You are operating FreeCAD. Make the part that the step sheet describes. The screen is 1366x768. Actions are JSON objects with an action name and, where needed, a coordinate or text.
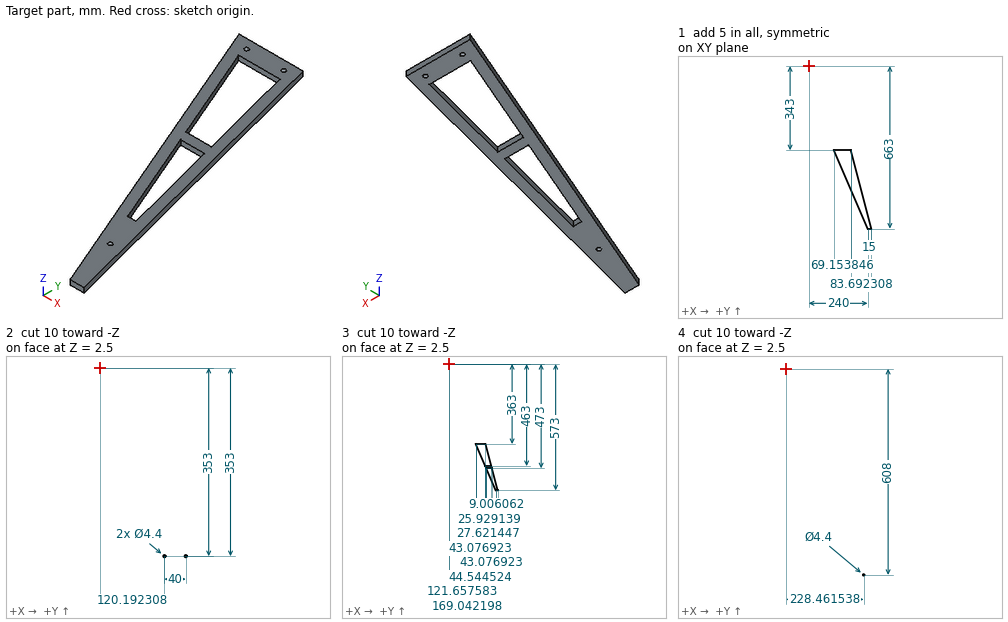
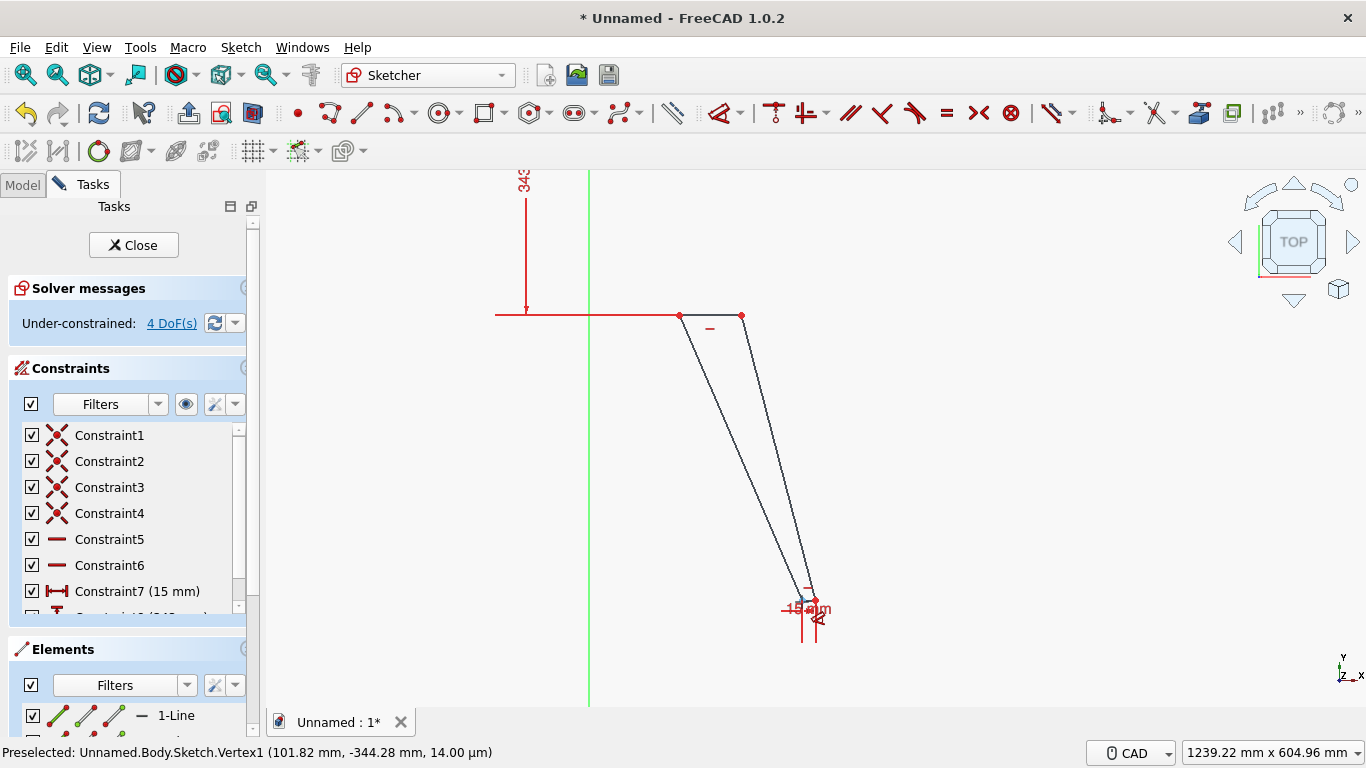
{"action": "left_click", "coordinate": [802, 601]}
{"action": "left_click", "coordinate": [696, 635]}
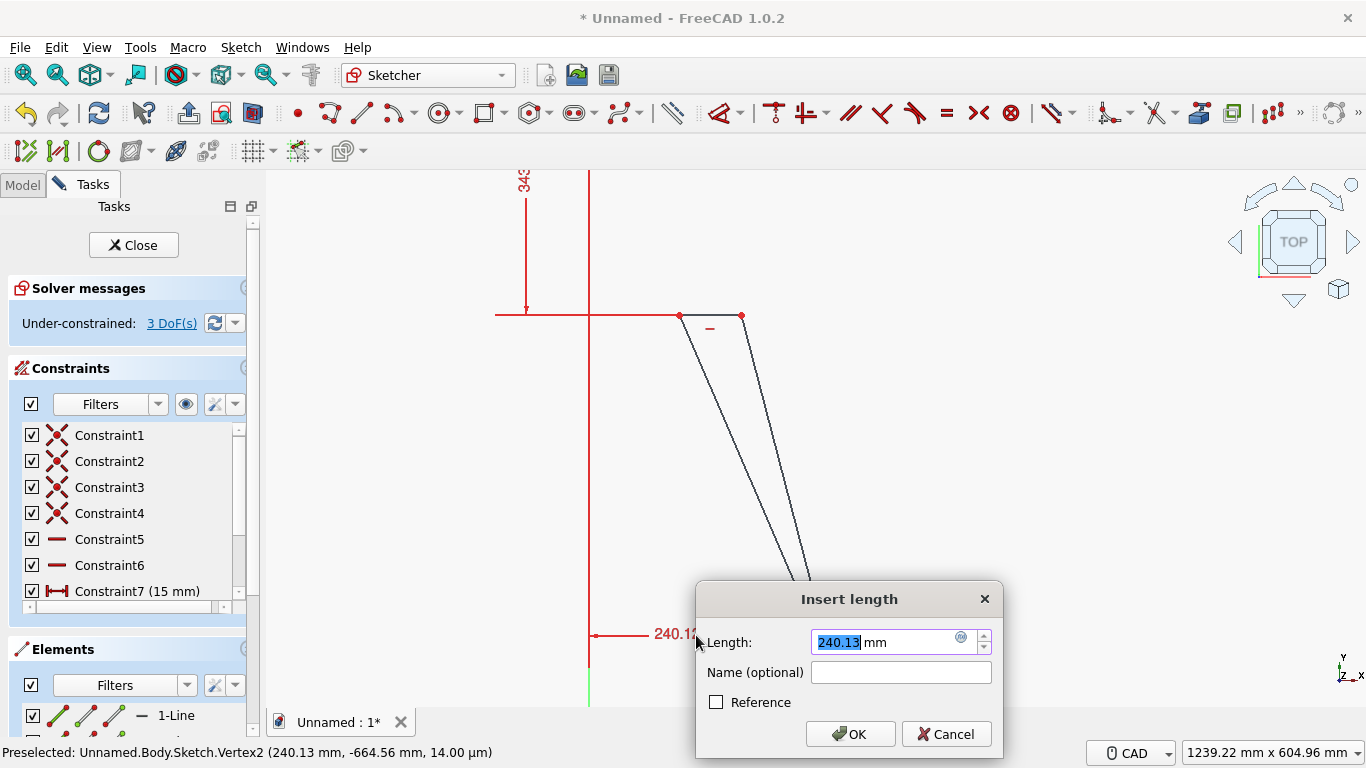
{"action": "type", "text": "240"}
{"action": "key", "text": "Return"}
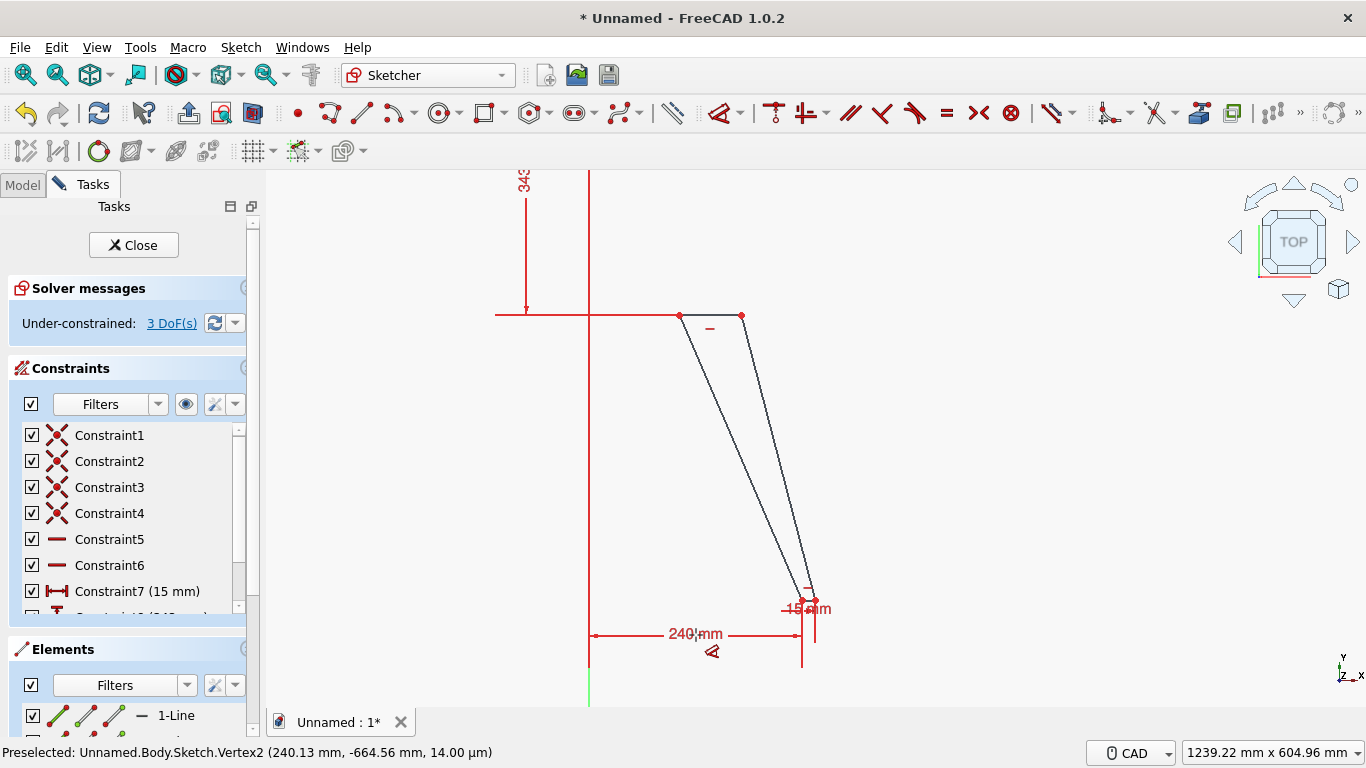
{"action": "left_click", "coordinate": [802, 601]}
{"action": "left_click", "coordinate": [555, 399]}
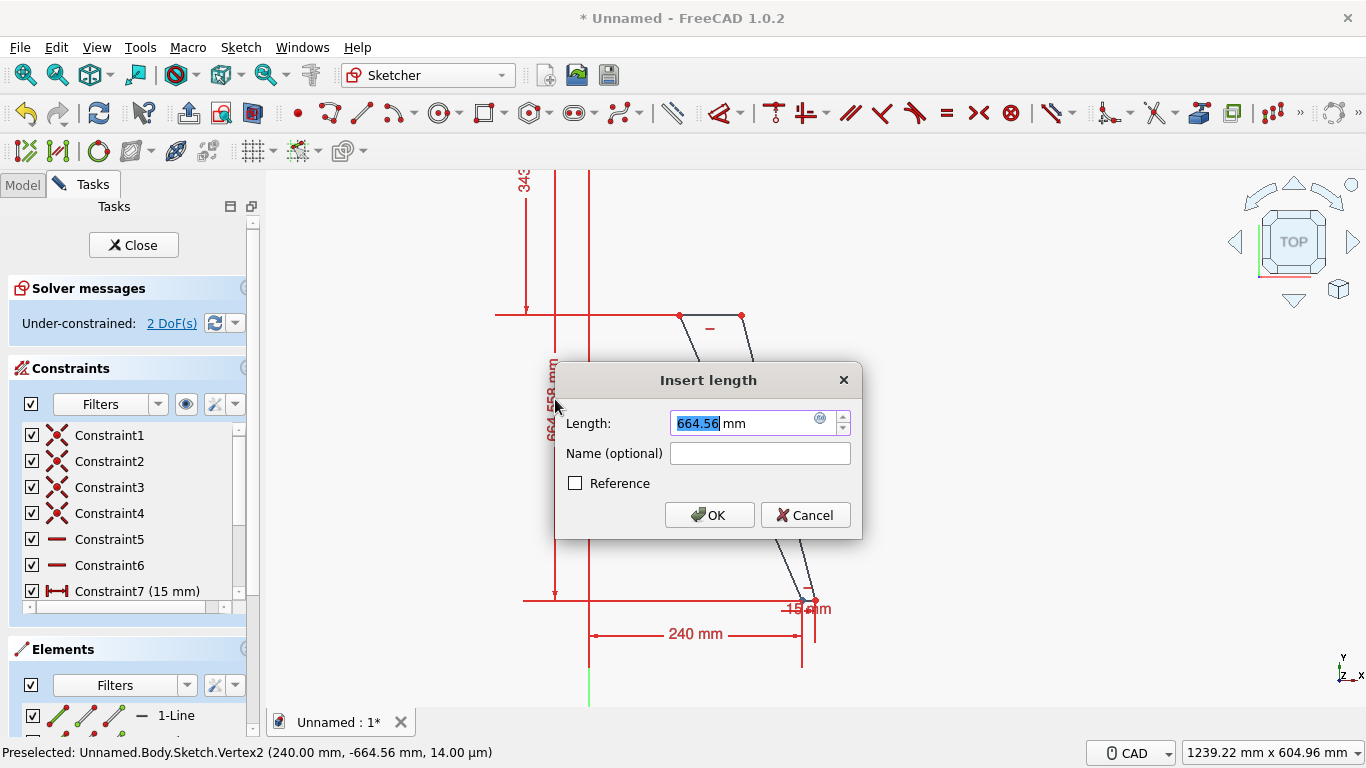
{"action": "type", "text": "663"}
{"action": "key", "text": "Return"}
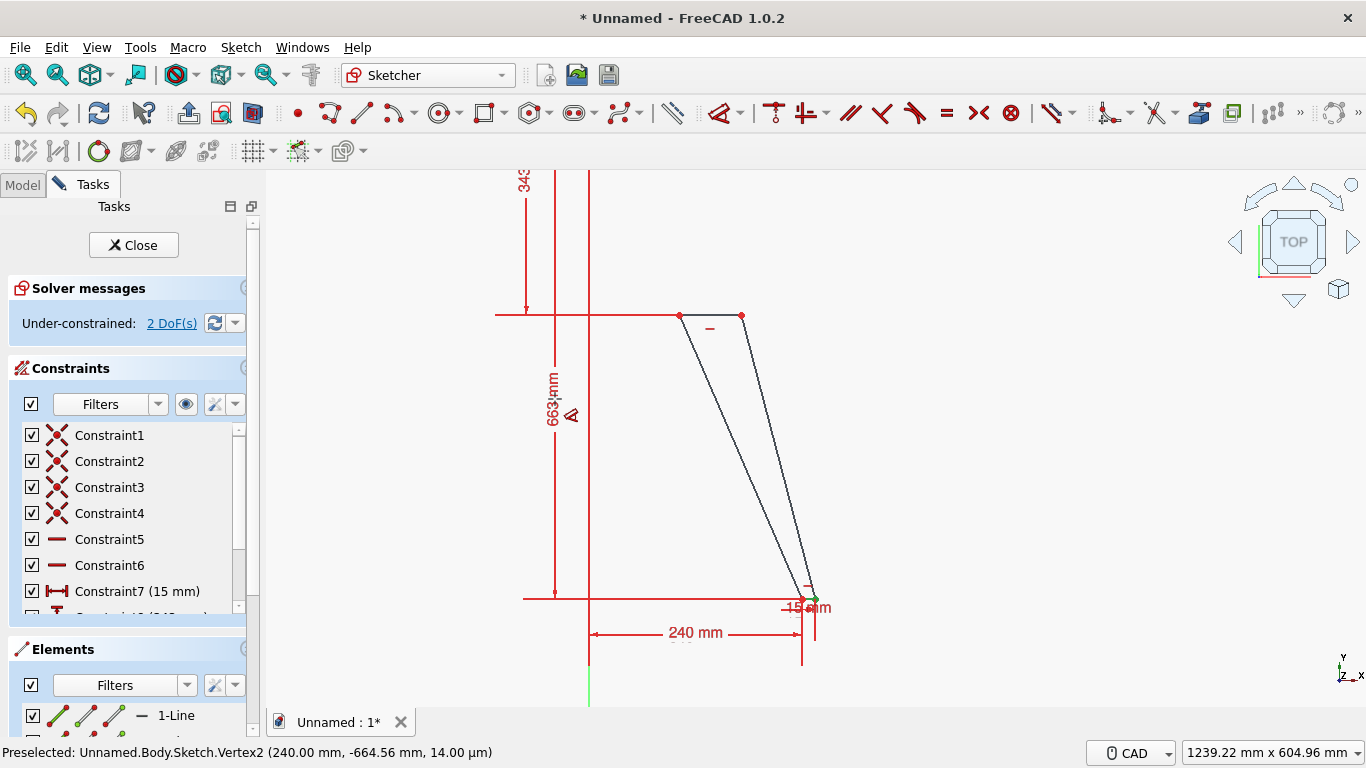
{"action": "left_click", "coordinate": [723, 315]}
{"action": "left_click", "coordinate": [710, 349]}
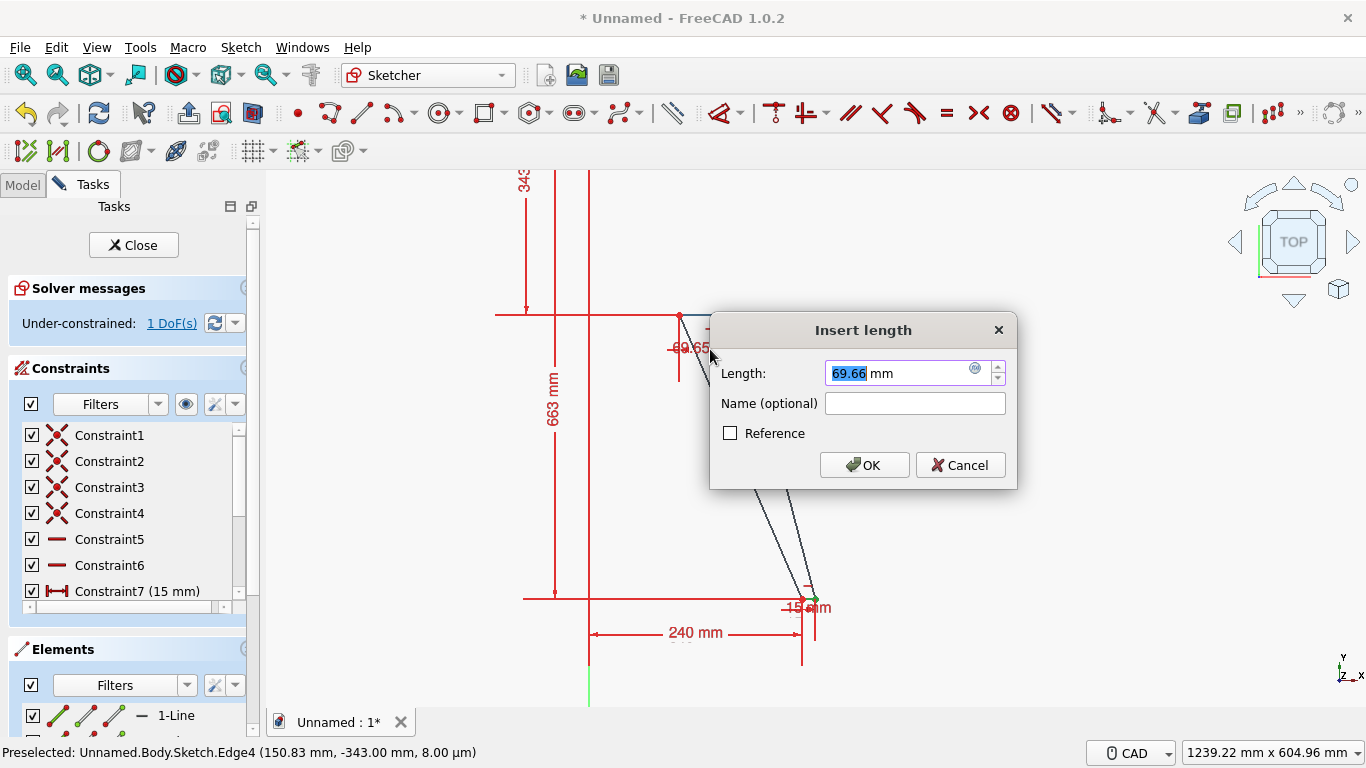
{"action": "type", "text": "69.153846"}
{"action": "key", "text": "Return"}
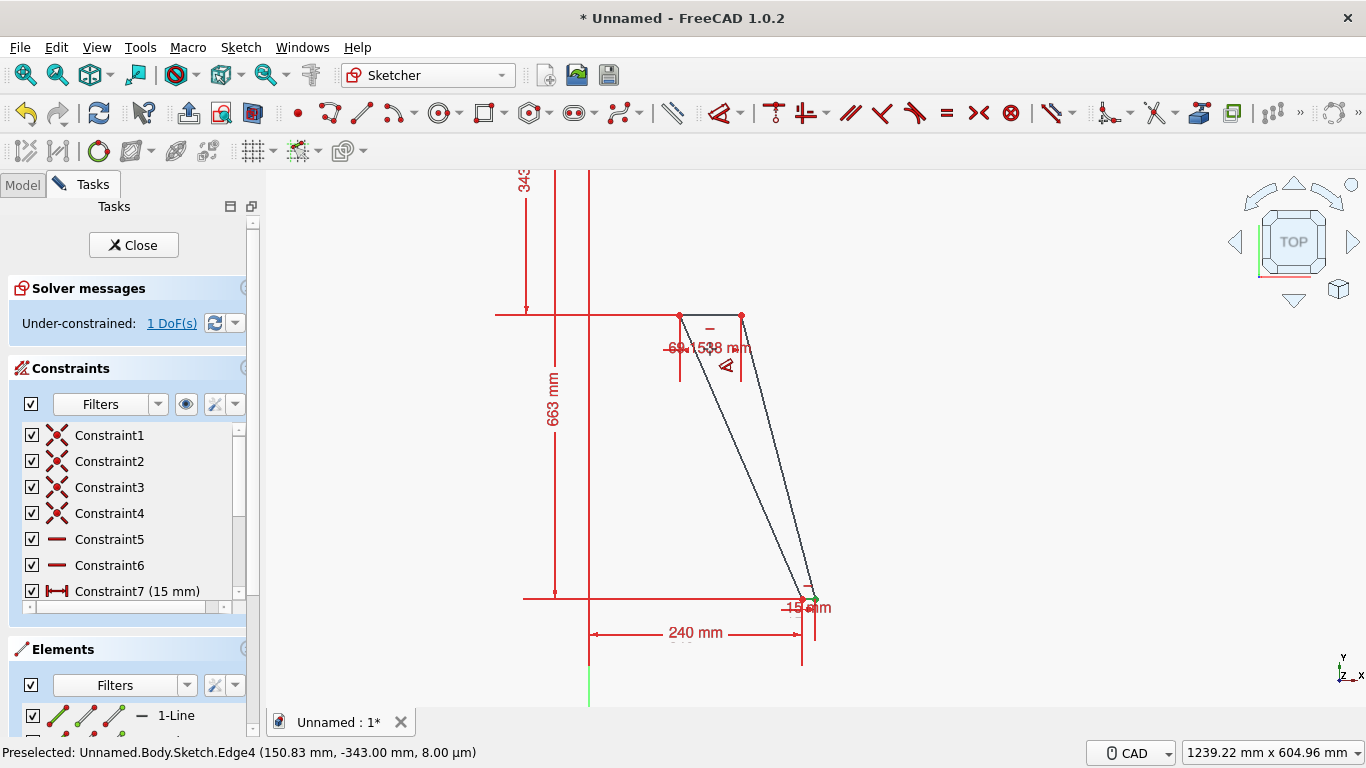
{"action": "left_click", "coordinate": [793, 514]}
{"action": "left_click", "coordinate": [778, 633]}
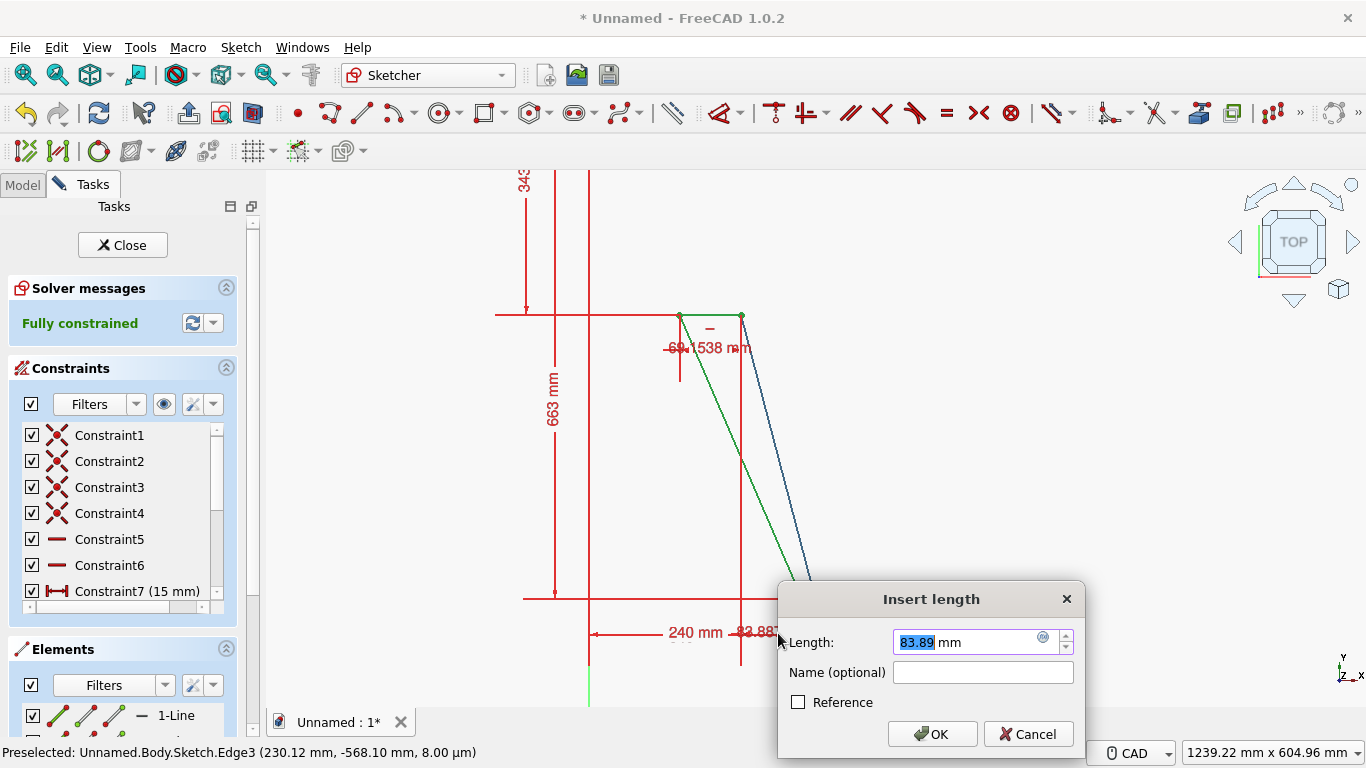
{"action": "type", "text": "83.692308"}
{"action": "key", "text": "Return"}
{"action": "key", "text": "Escape"}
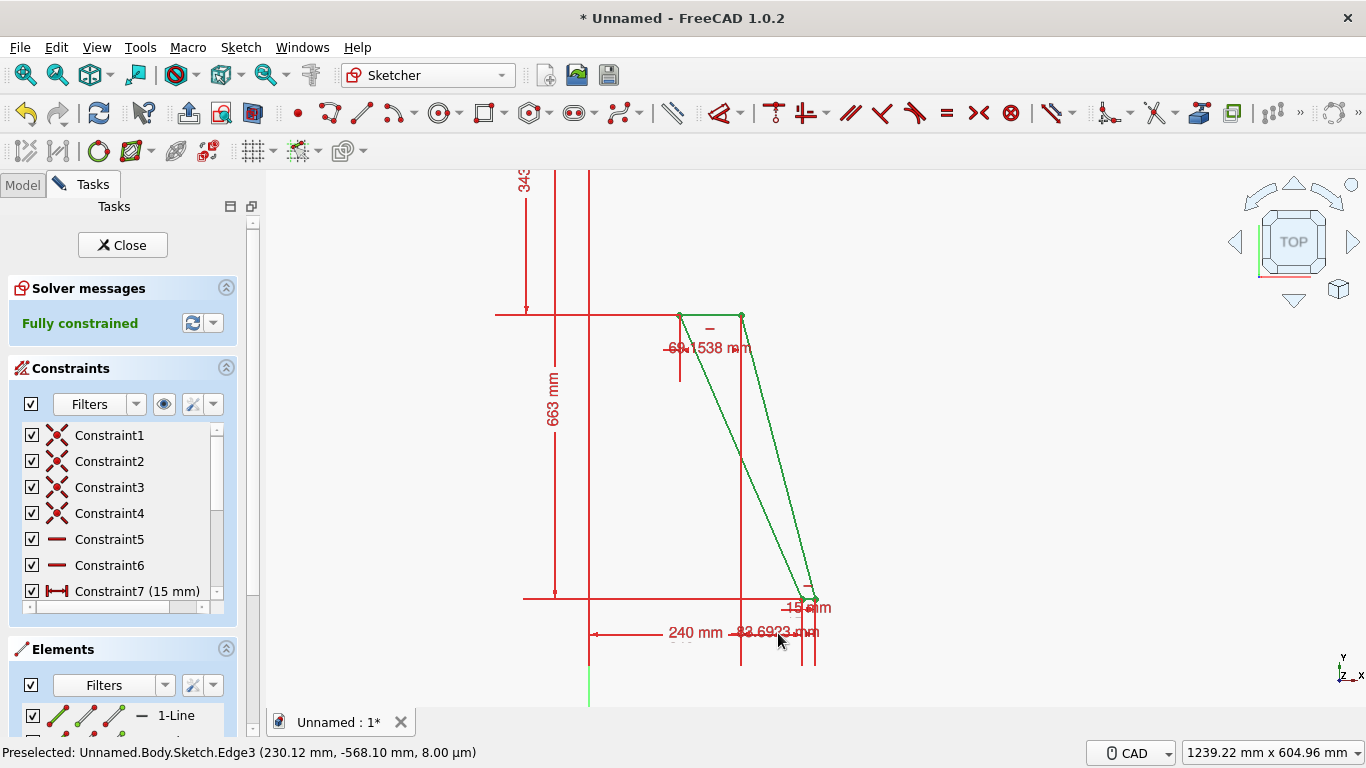
{"action": "left_click", "coordinate": [123, 245]}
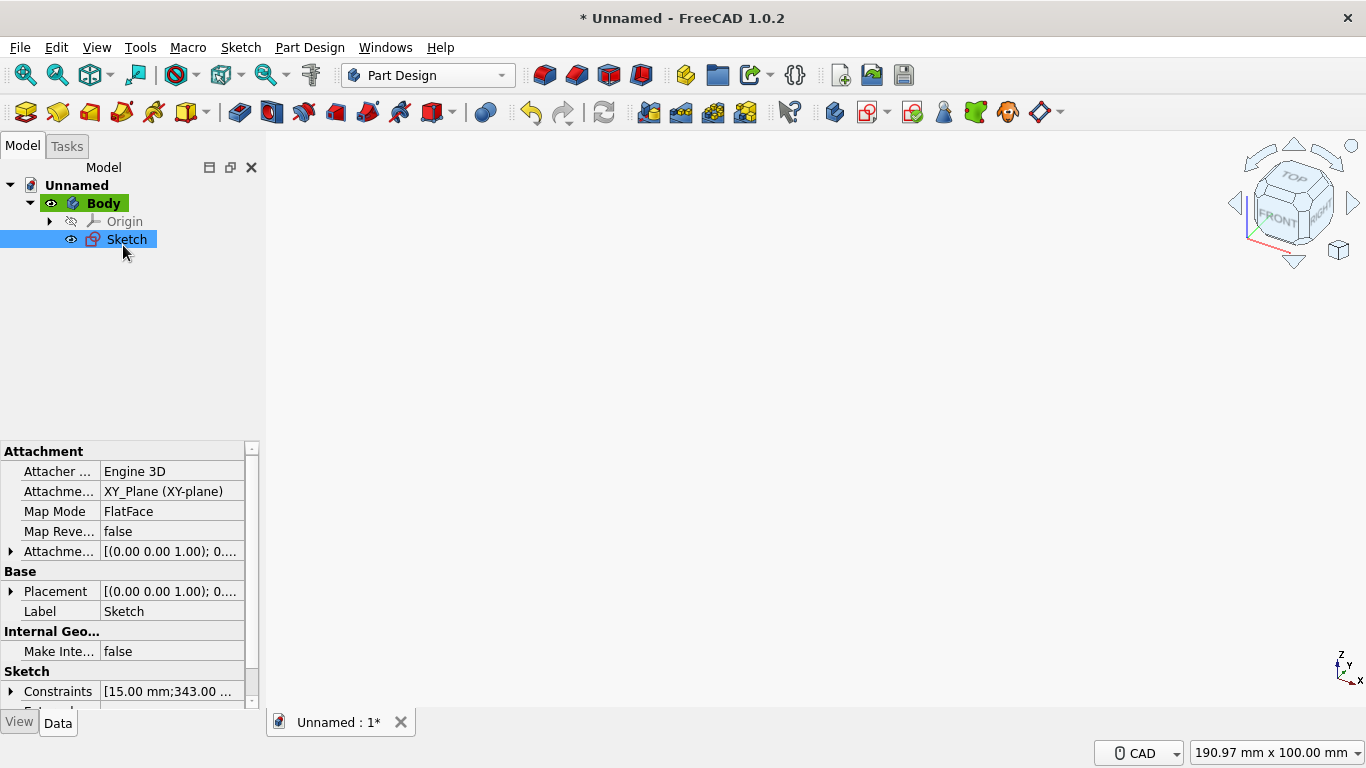
{"action": "left_click", "coordinate": [26, 112]}